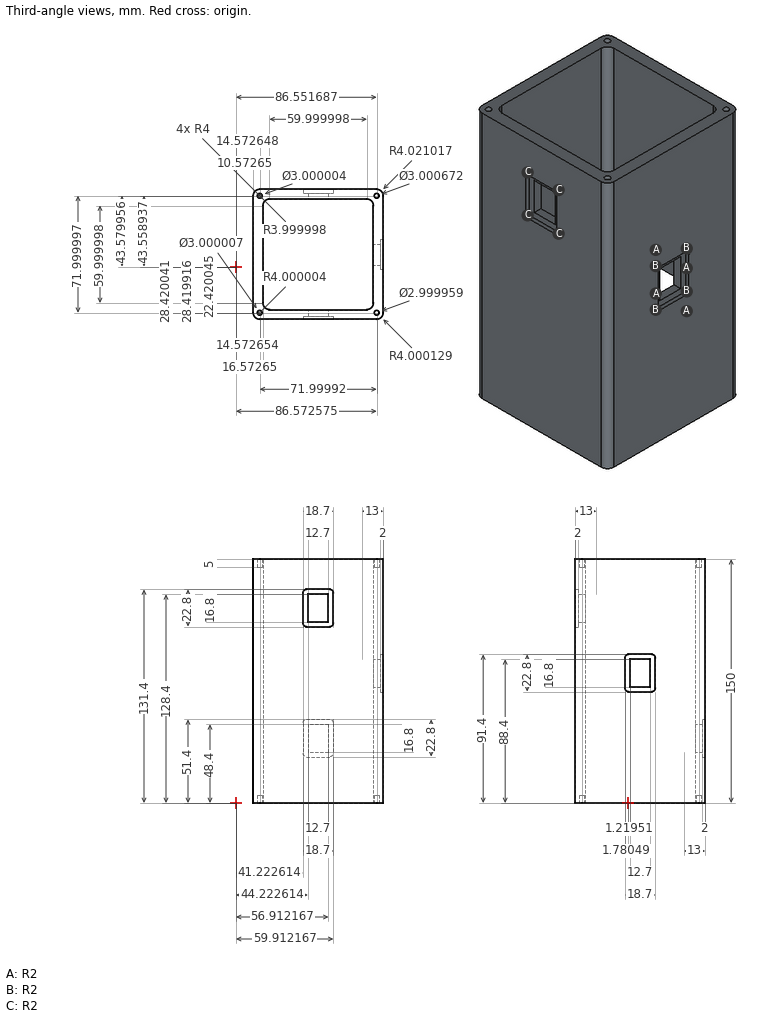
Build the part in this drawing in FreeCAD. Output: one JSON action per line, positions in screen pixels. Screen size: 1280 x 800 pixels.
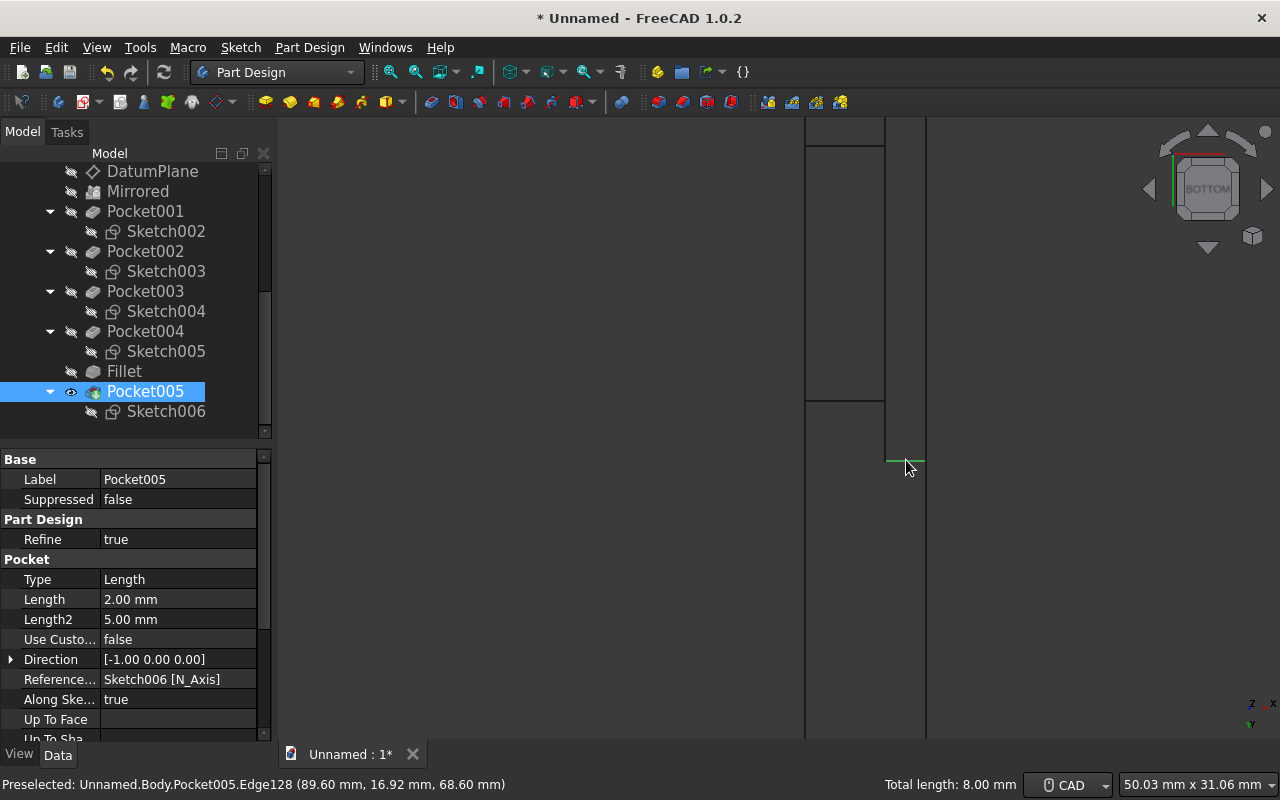
{"action": "key", "text": "v 1"}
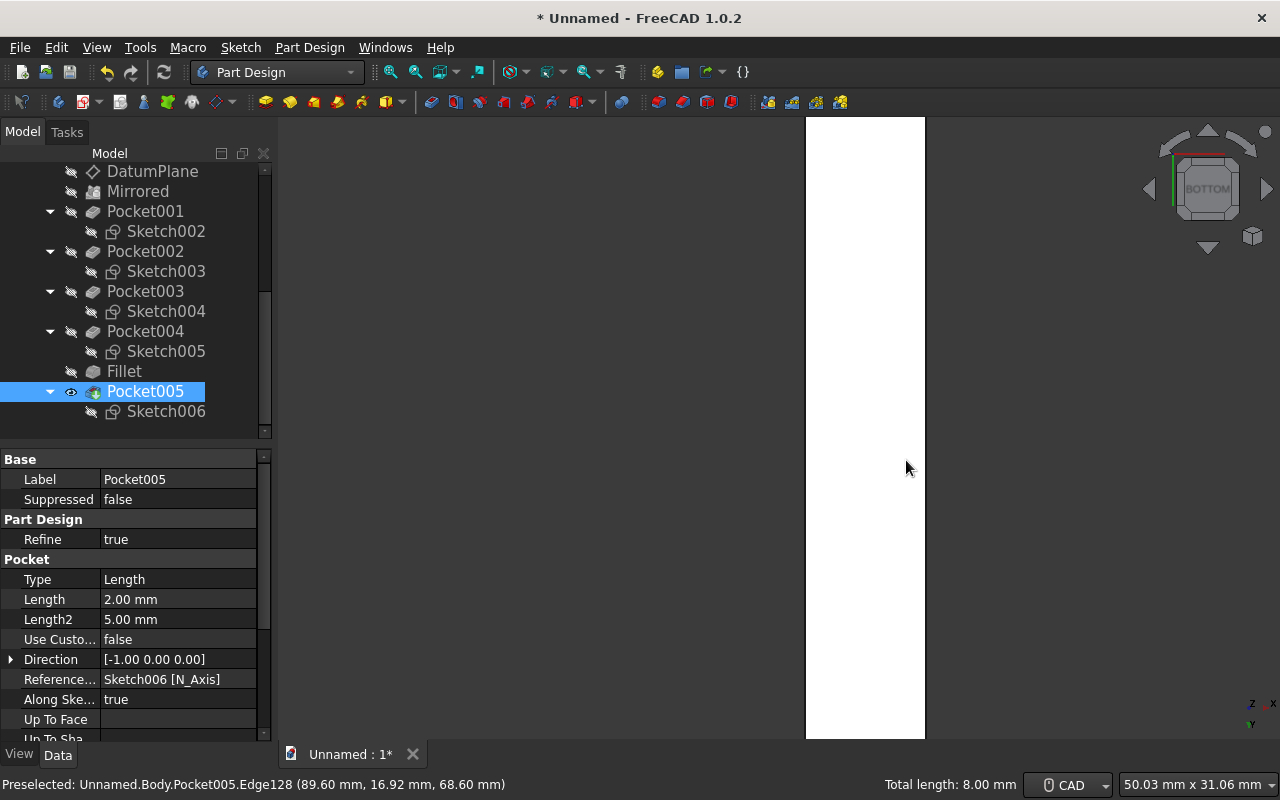
{"action": "left_click", "coordinate": [660, 102]}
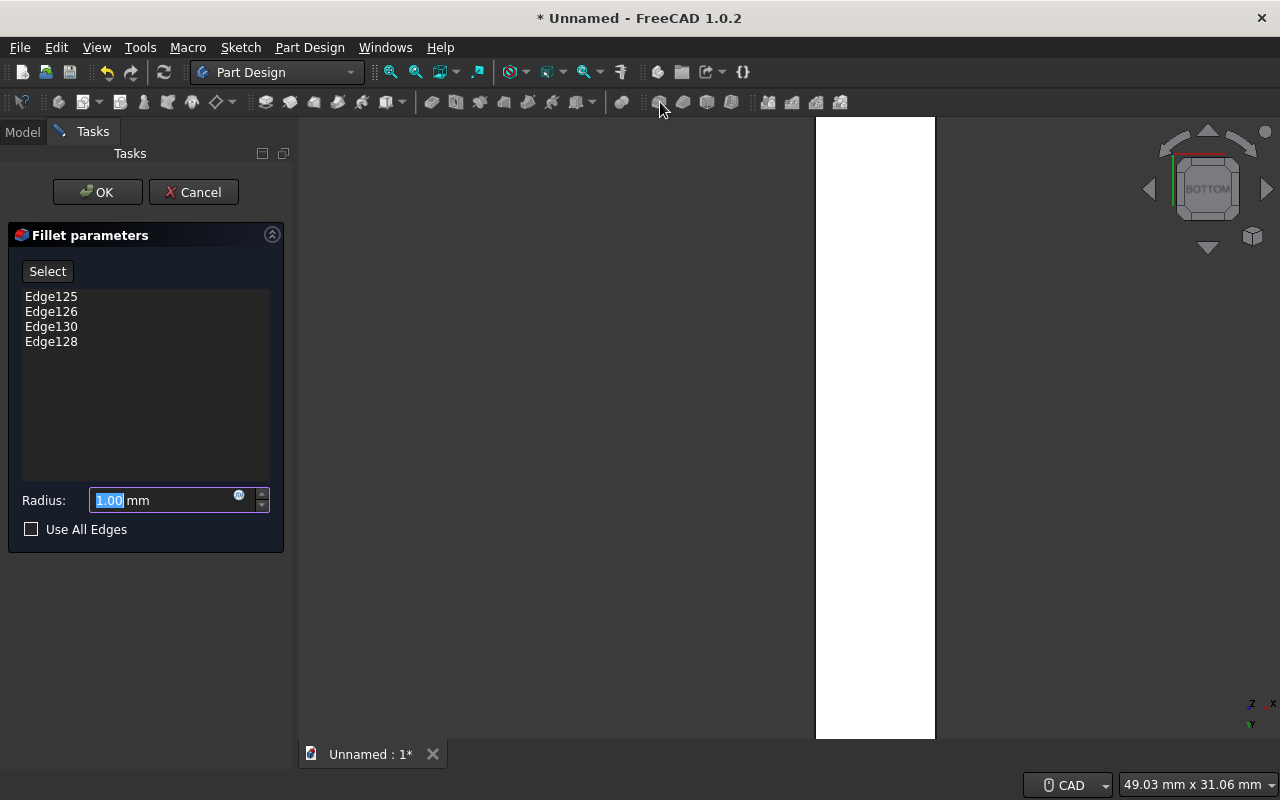
{"action": "type", "text": "2"}
{"action": "key", "text": "Tab"}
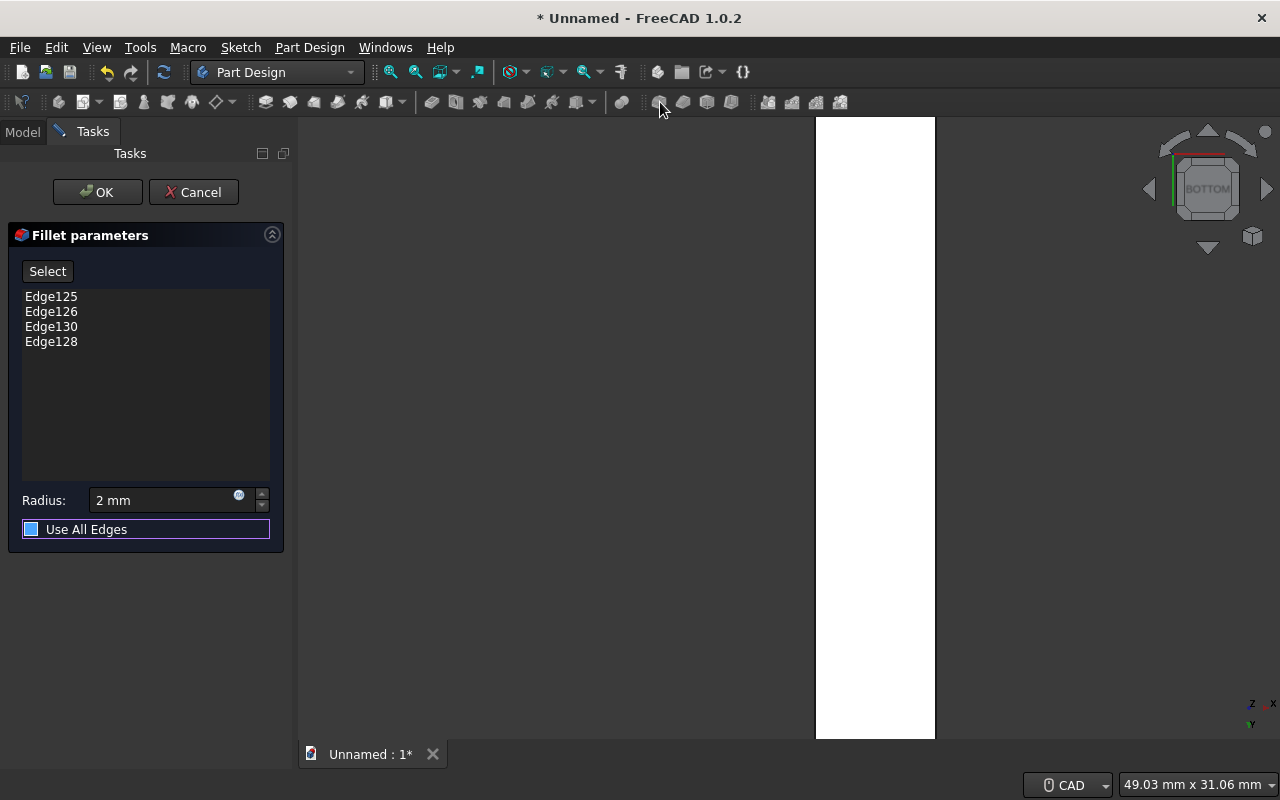
{"action": "left_click", "coordinate": [98, 192]}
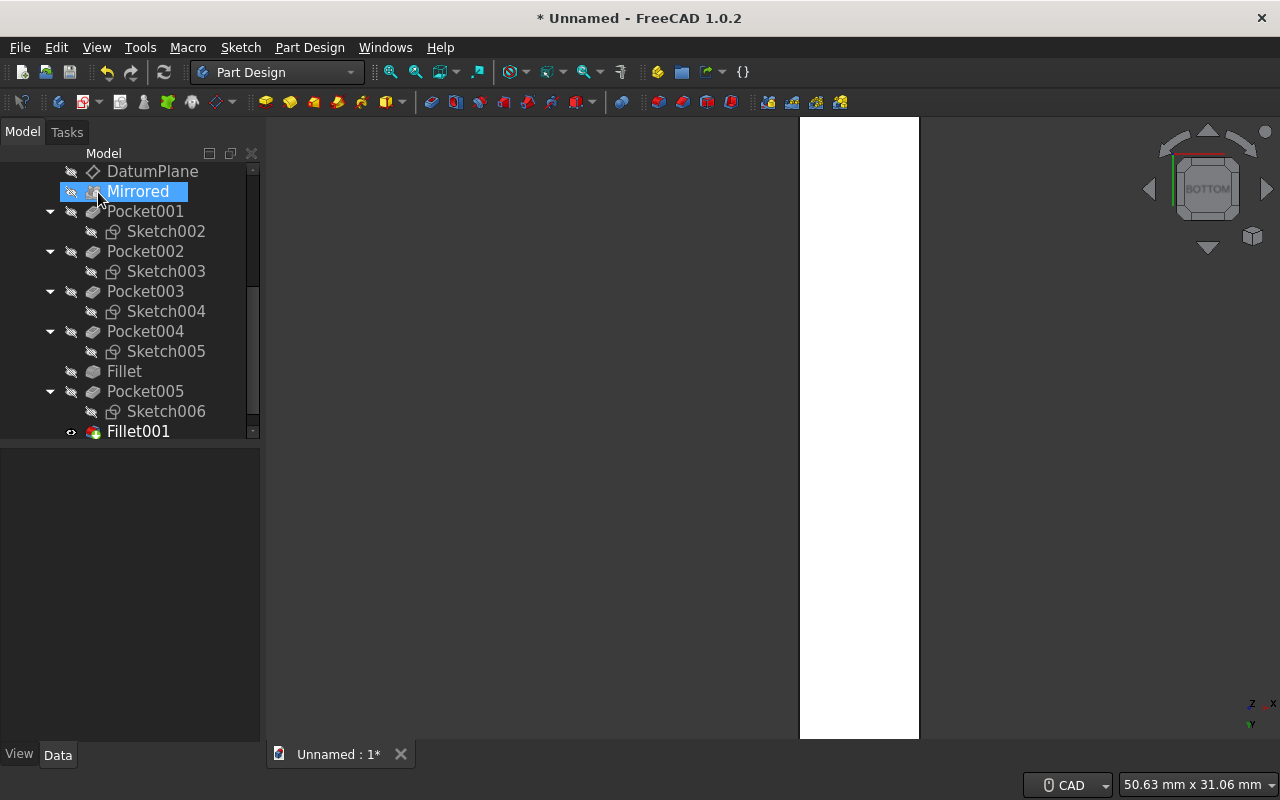
{"action": "key", "text": "v f"}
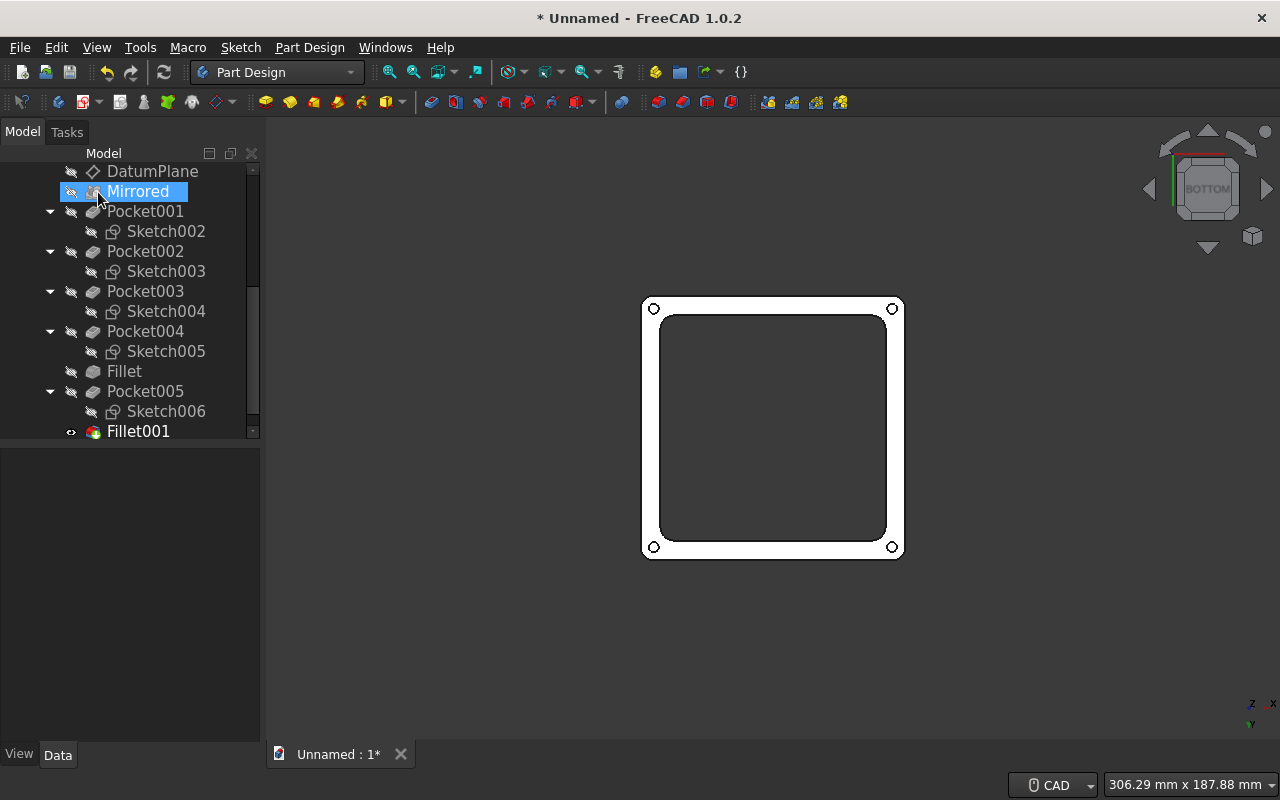
{"action": "key", "text": "0"}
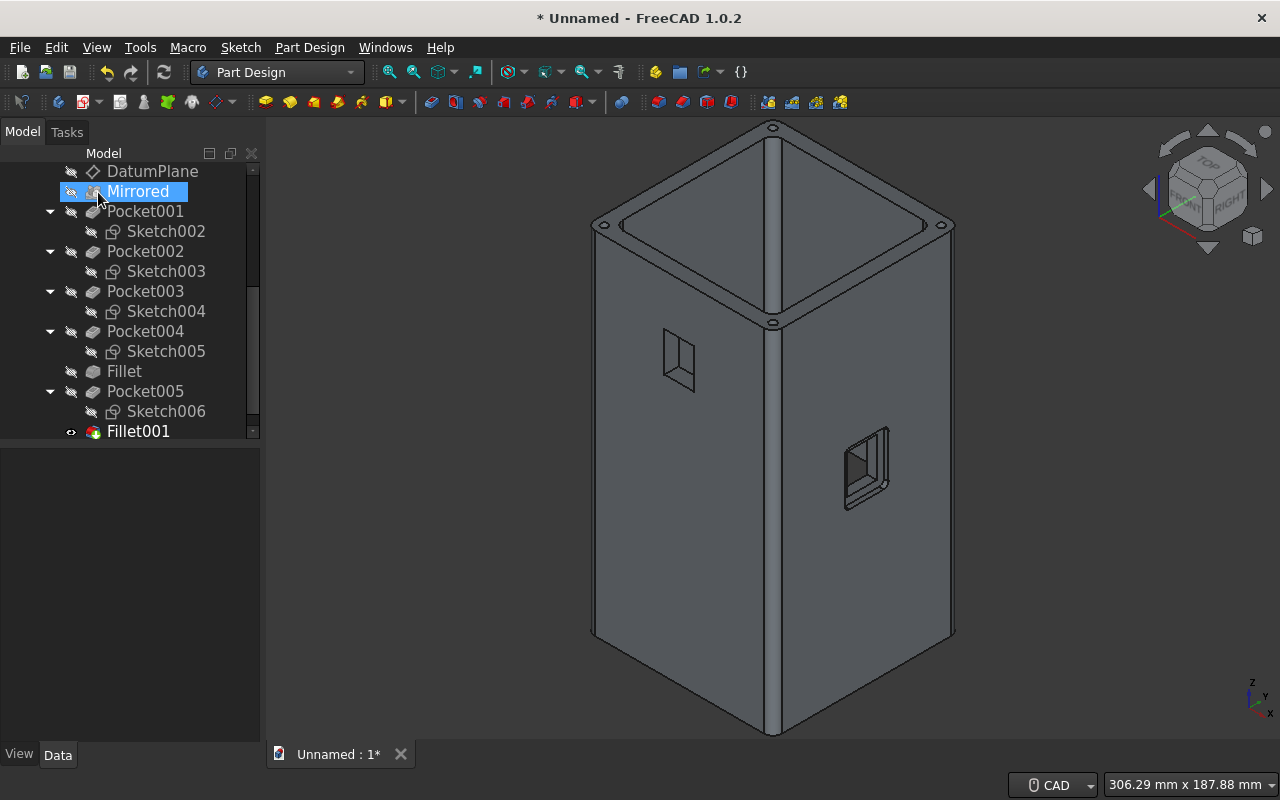
{"action": "left_click", "coordinate": [390, 72]}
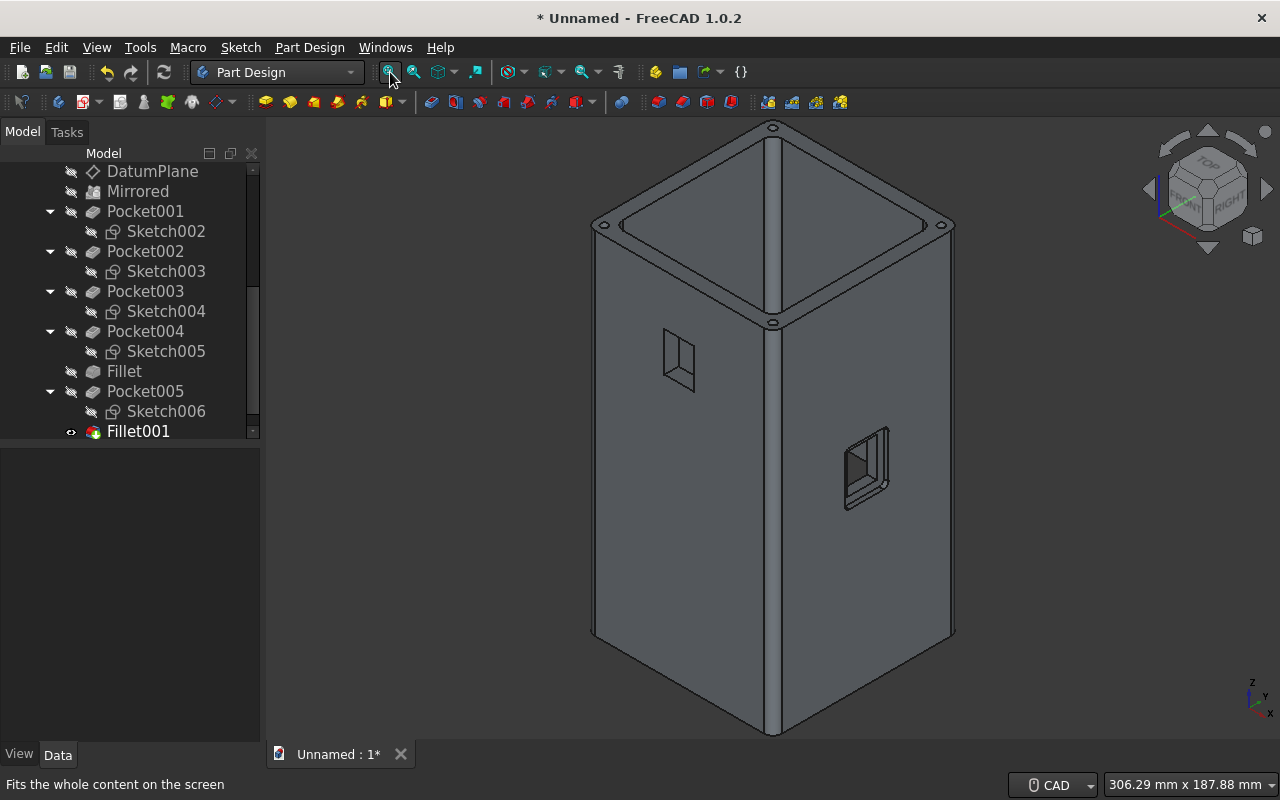
{"action": "left_click", "coordinate": [679, 481]}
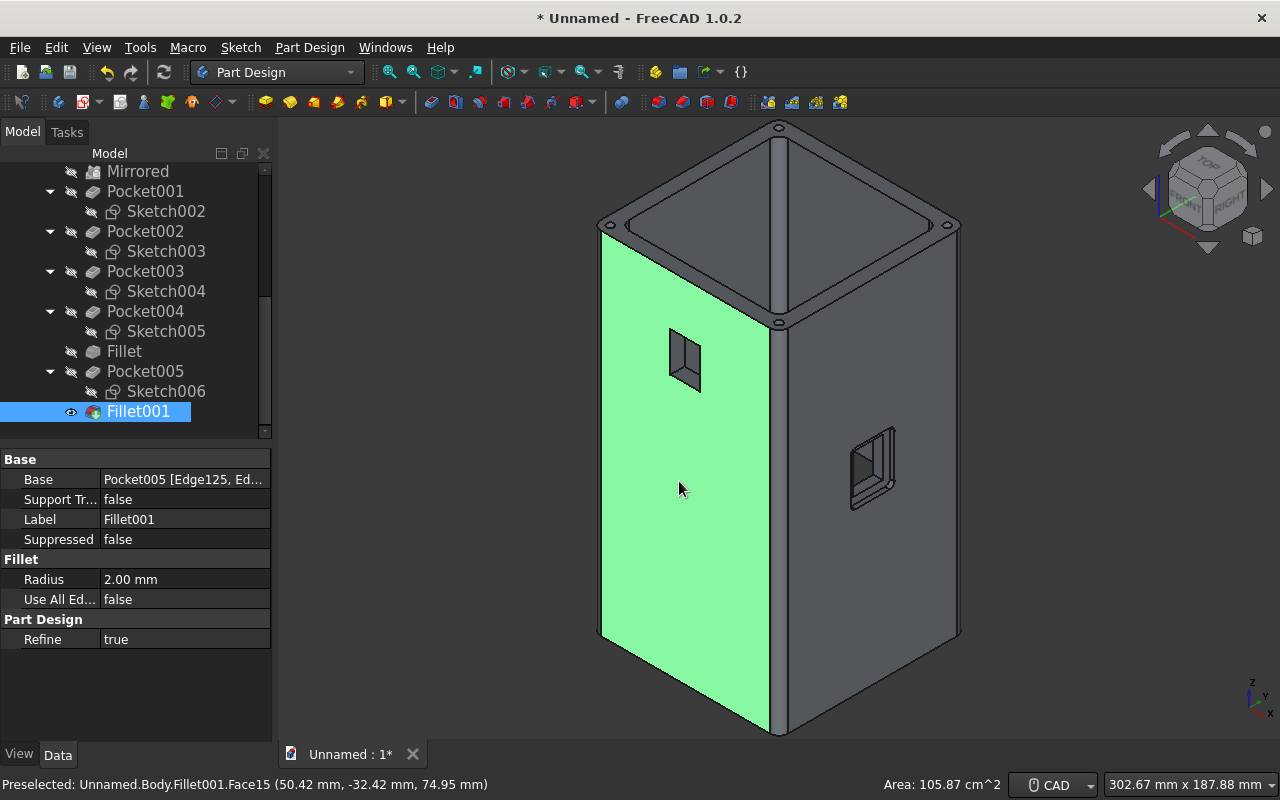
{"action": "left_click", "coordinate": [84, 102]}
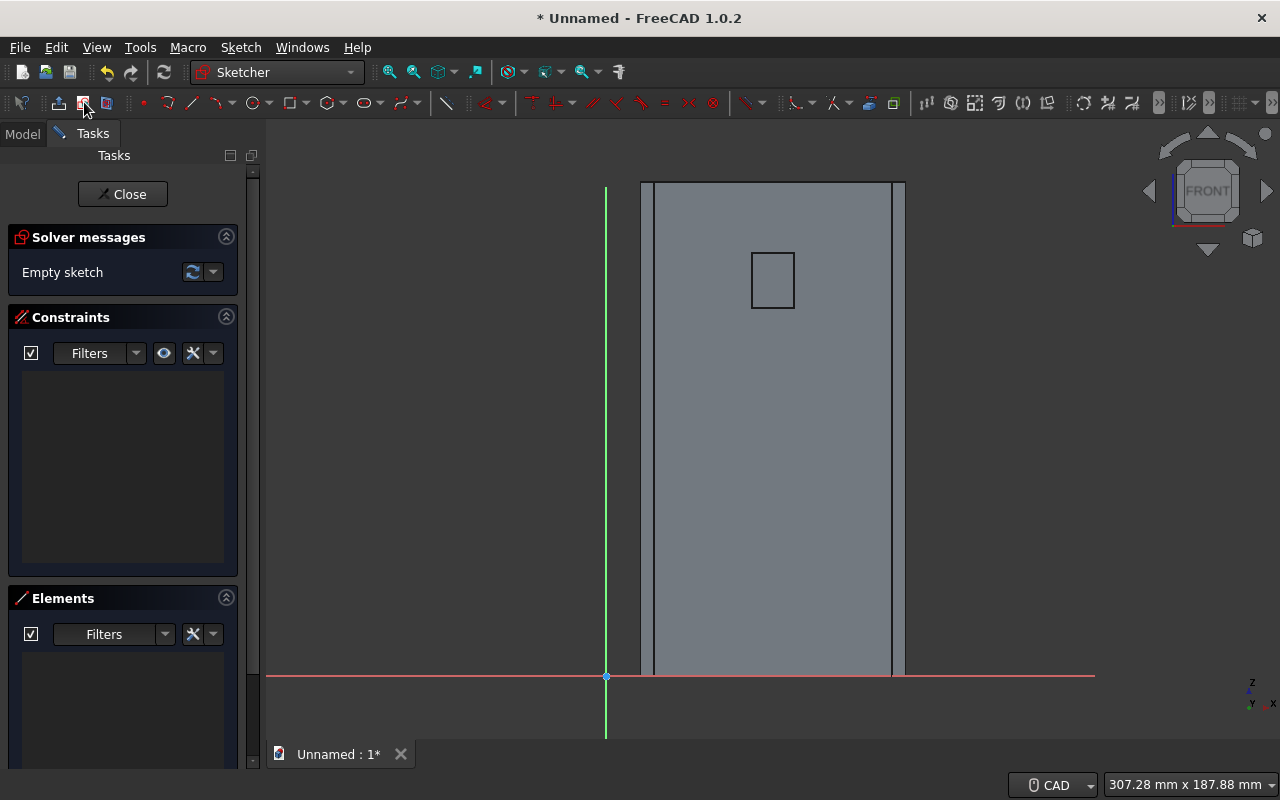
{"action": "scroll", "coordinate": [790, 243], "scroll_direction": "up", "scroll_amount": 8}